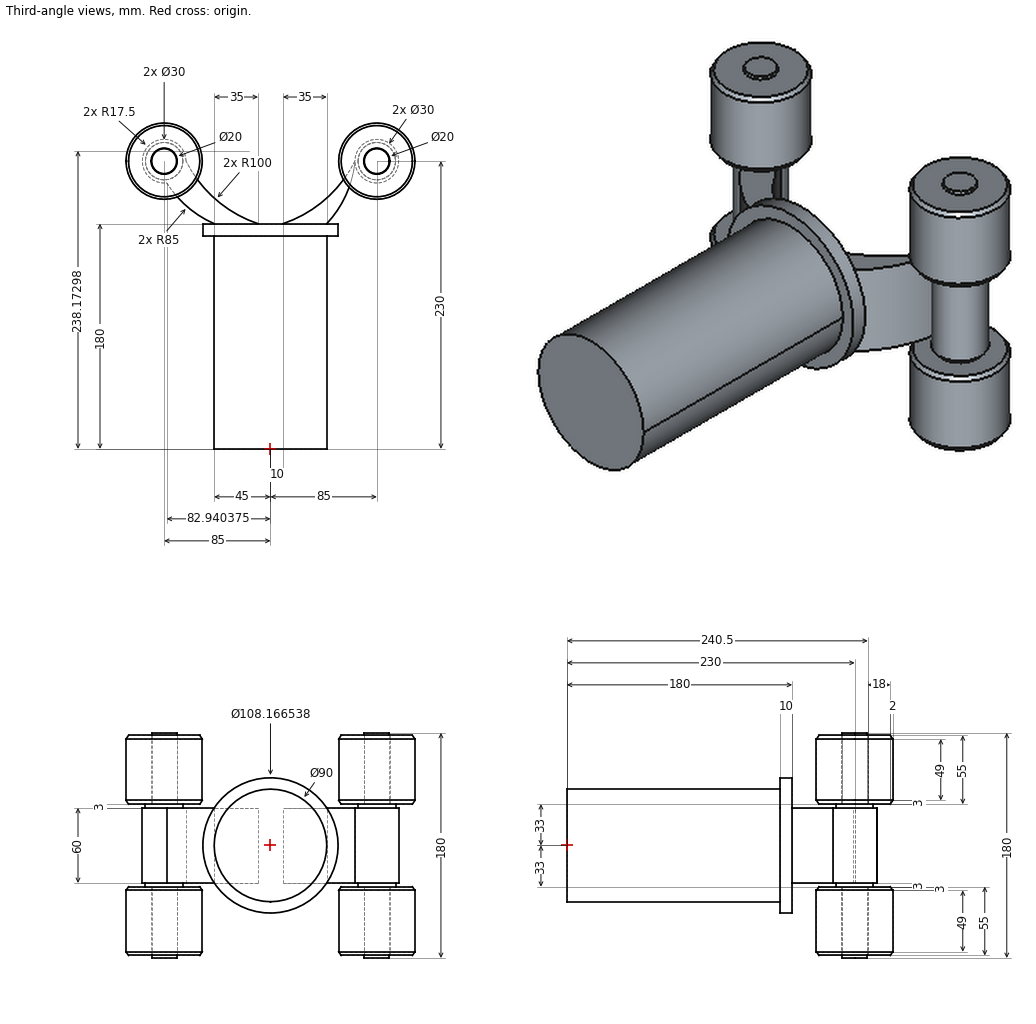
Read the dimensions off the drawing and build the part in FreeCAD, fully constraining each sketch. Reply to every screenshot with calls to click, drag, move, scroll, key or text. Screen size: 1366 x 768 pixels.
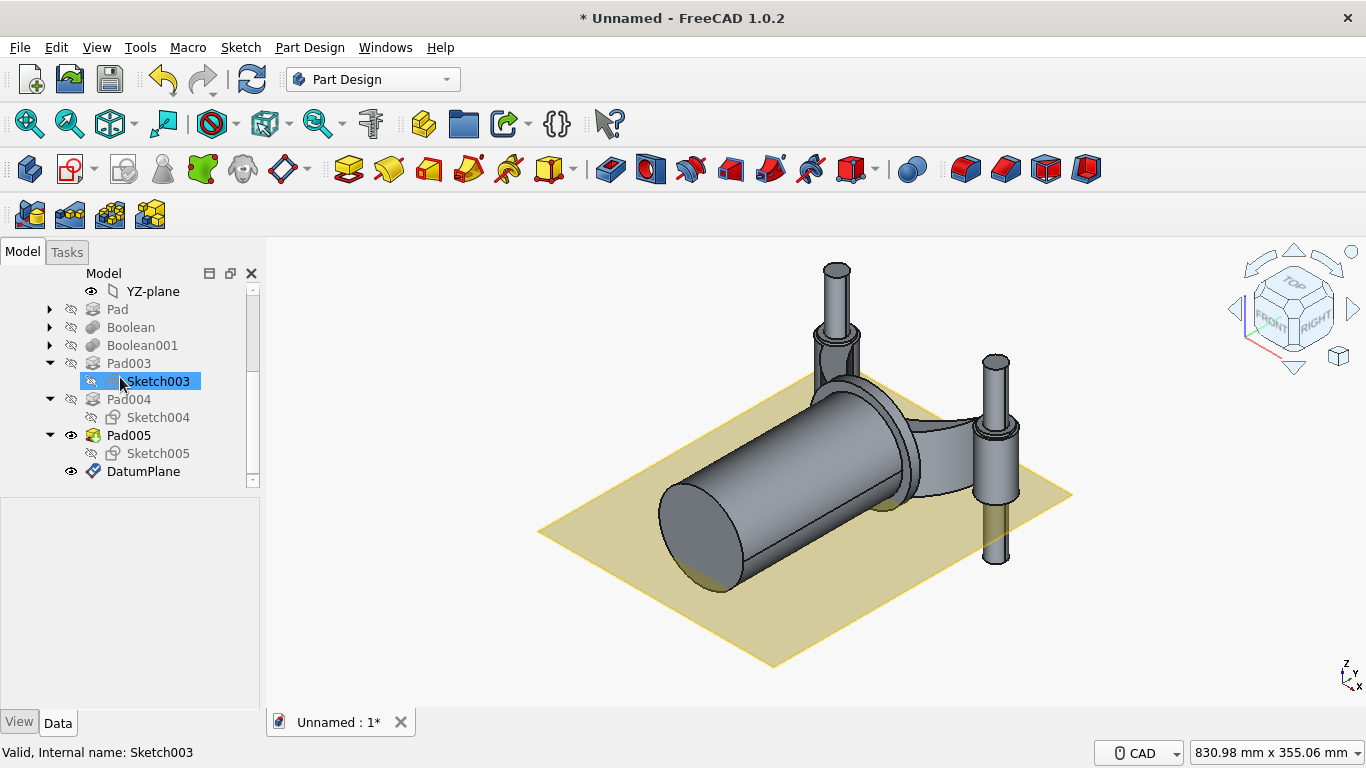
click(116, 471)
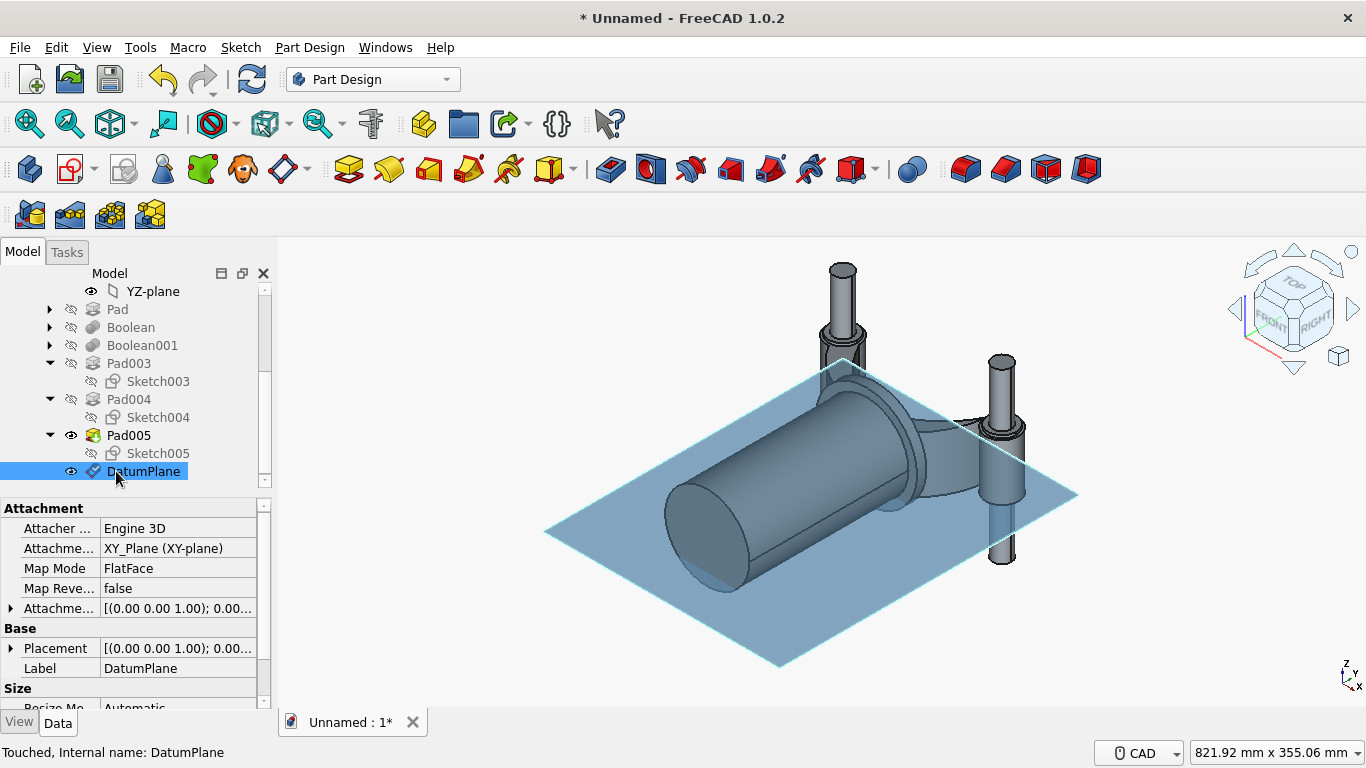
click(70, 170)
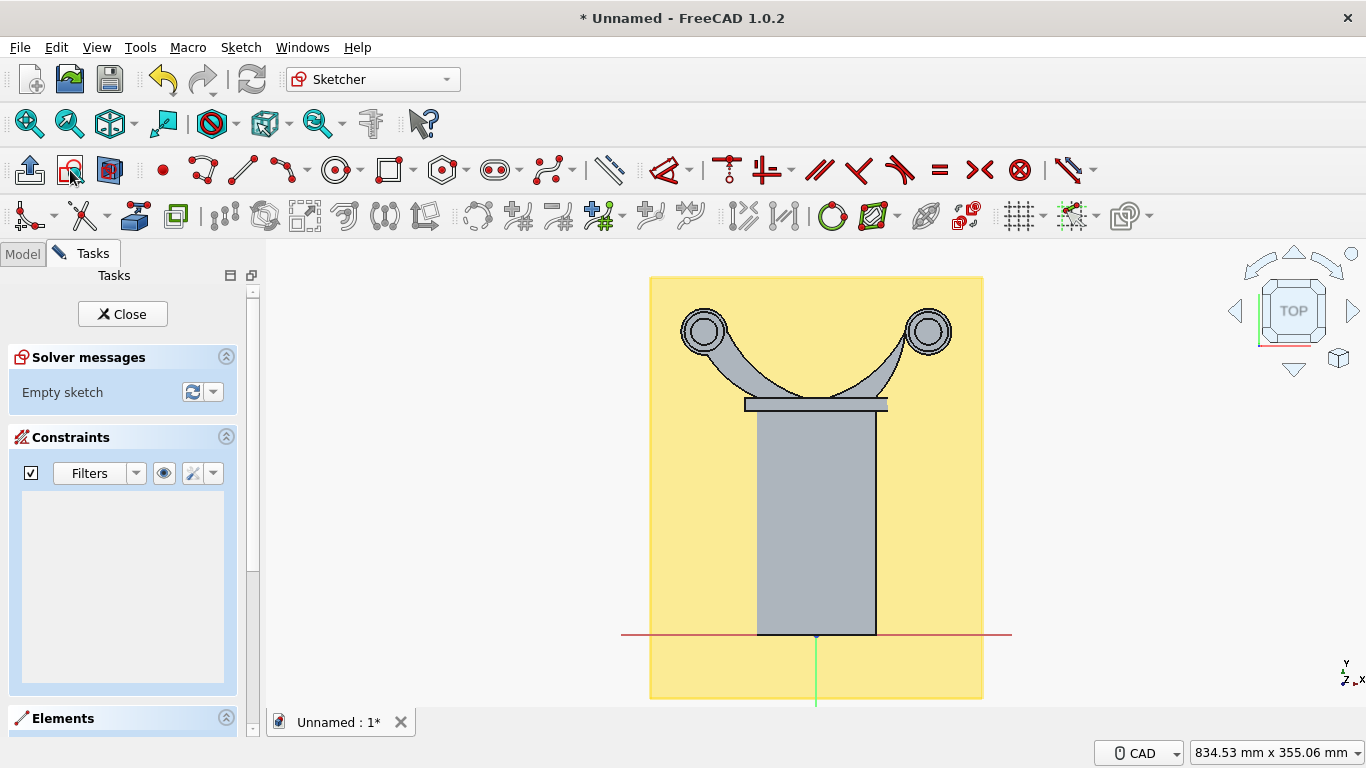
click(110, 170)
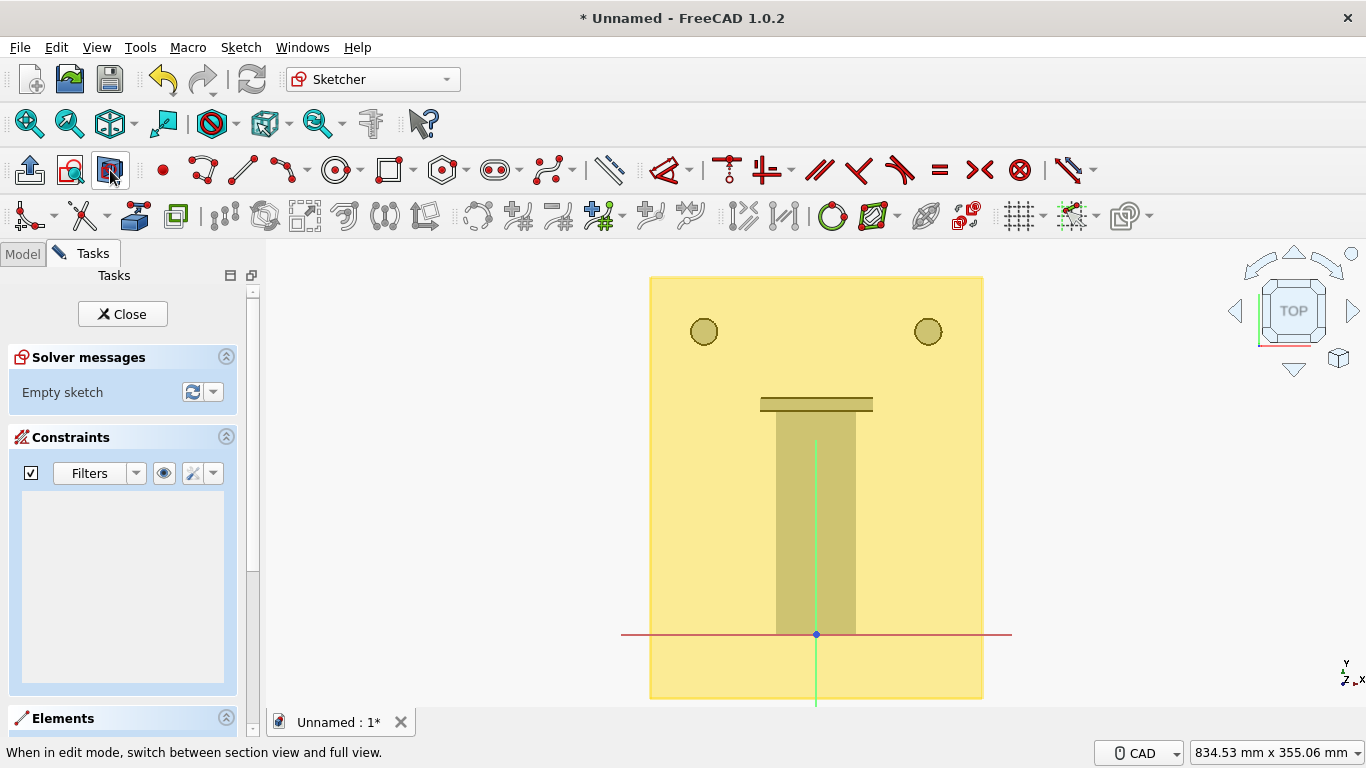
click(336, 170)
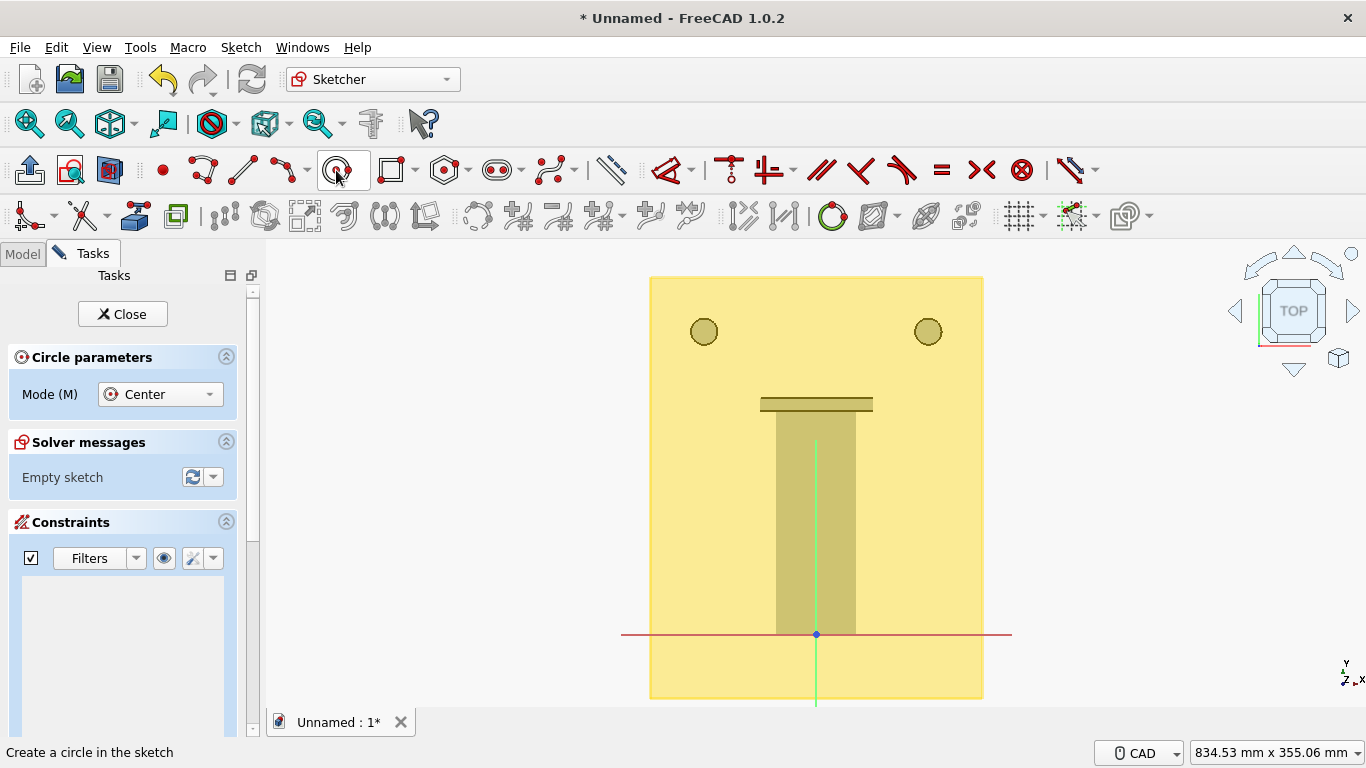
click(928, 332)
click(942, 318)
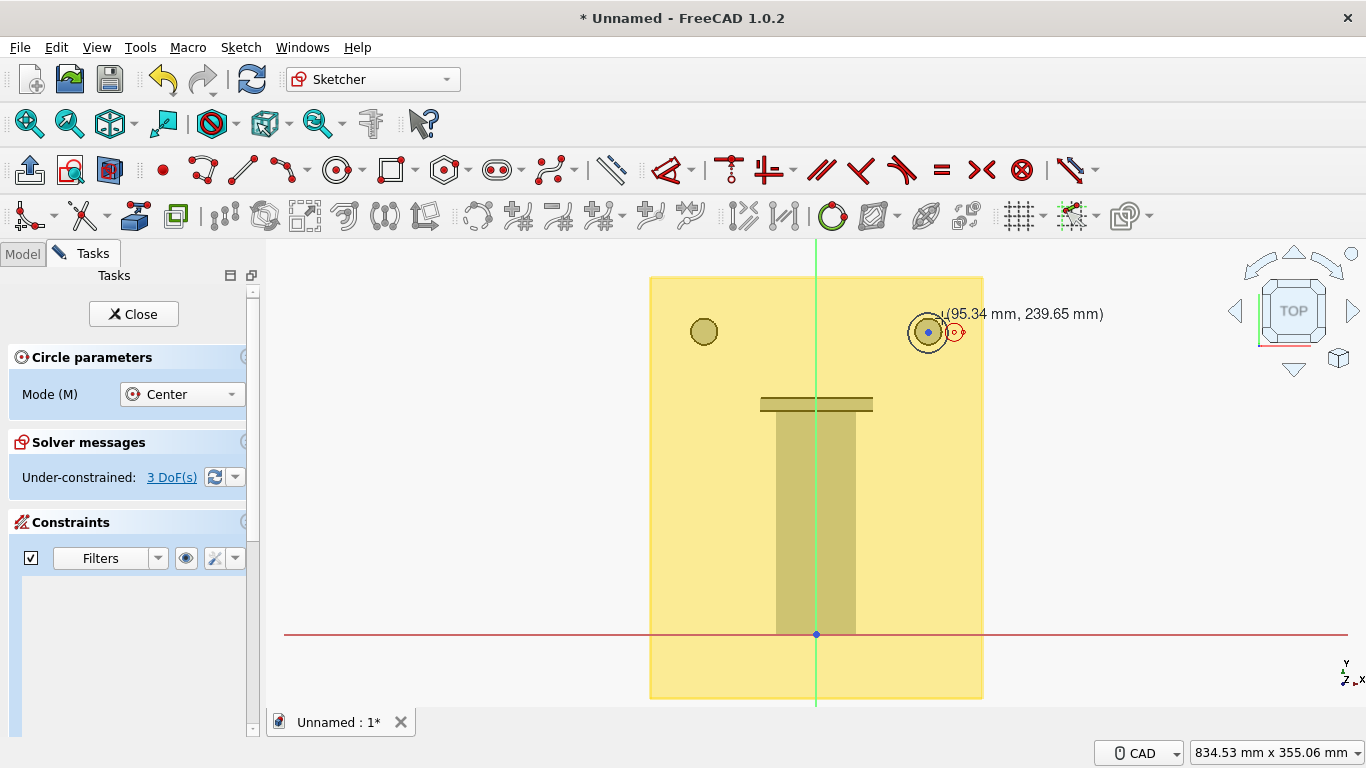
click(704, 332)
click(718, 318)
key(Escape)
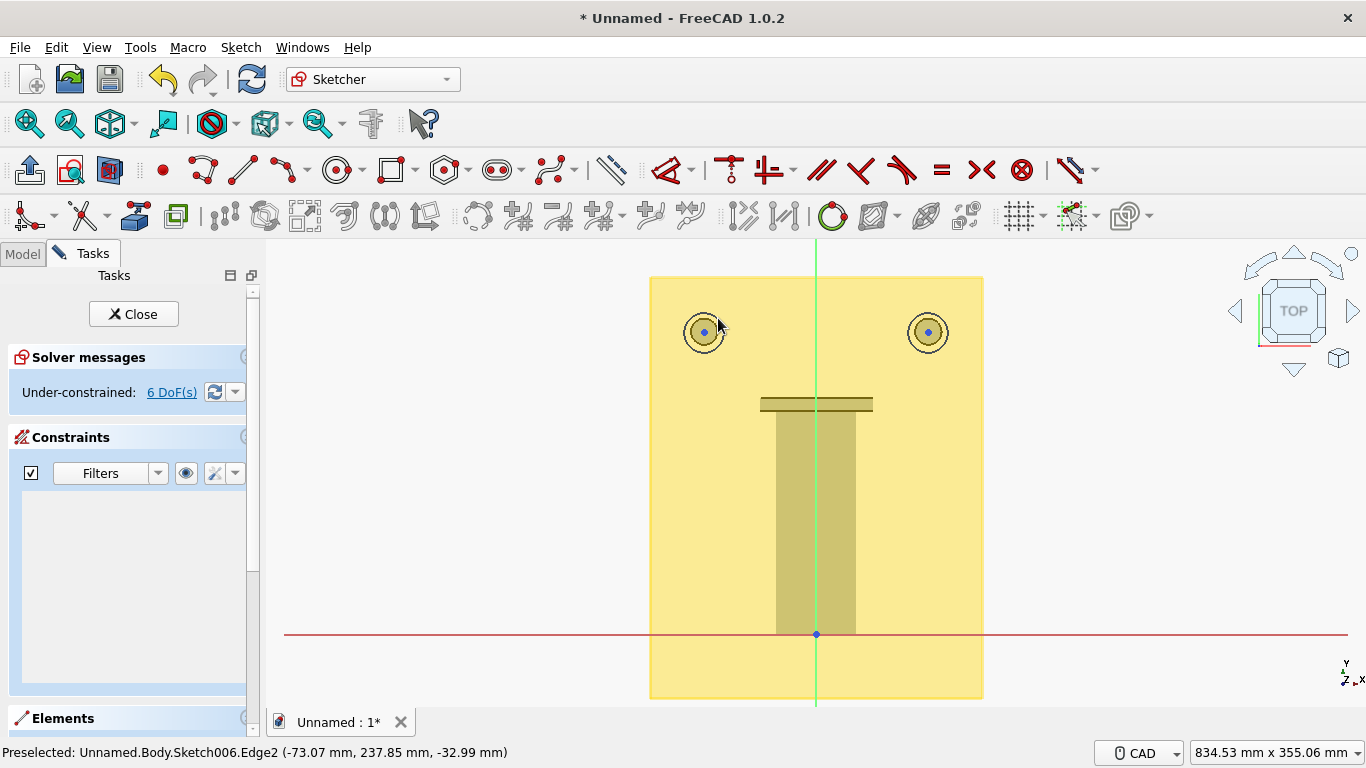
click(942, 319)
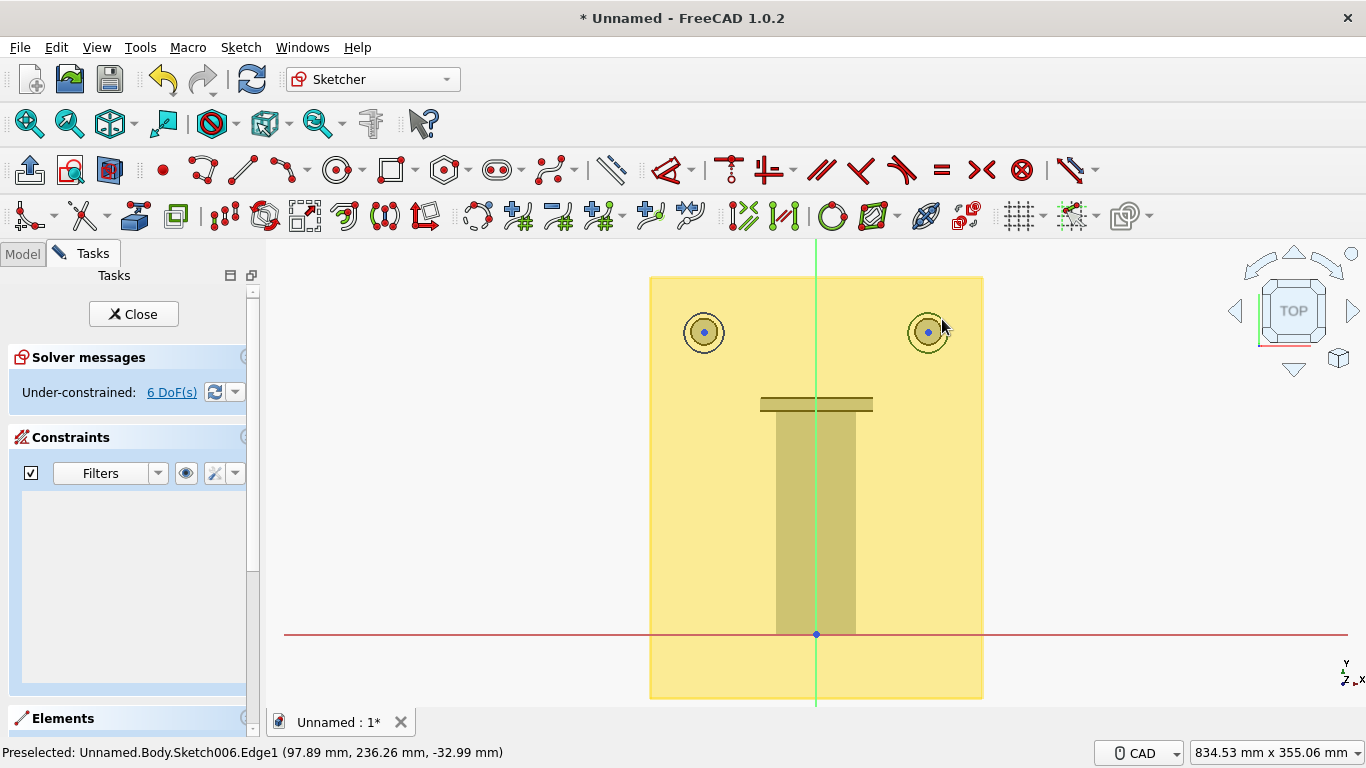
click(718, 319)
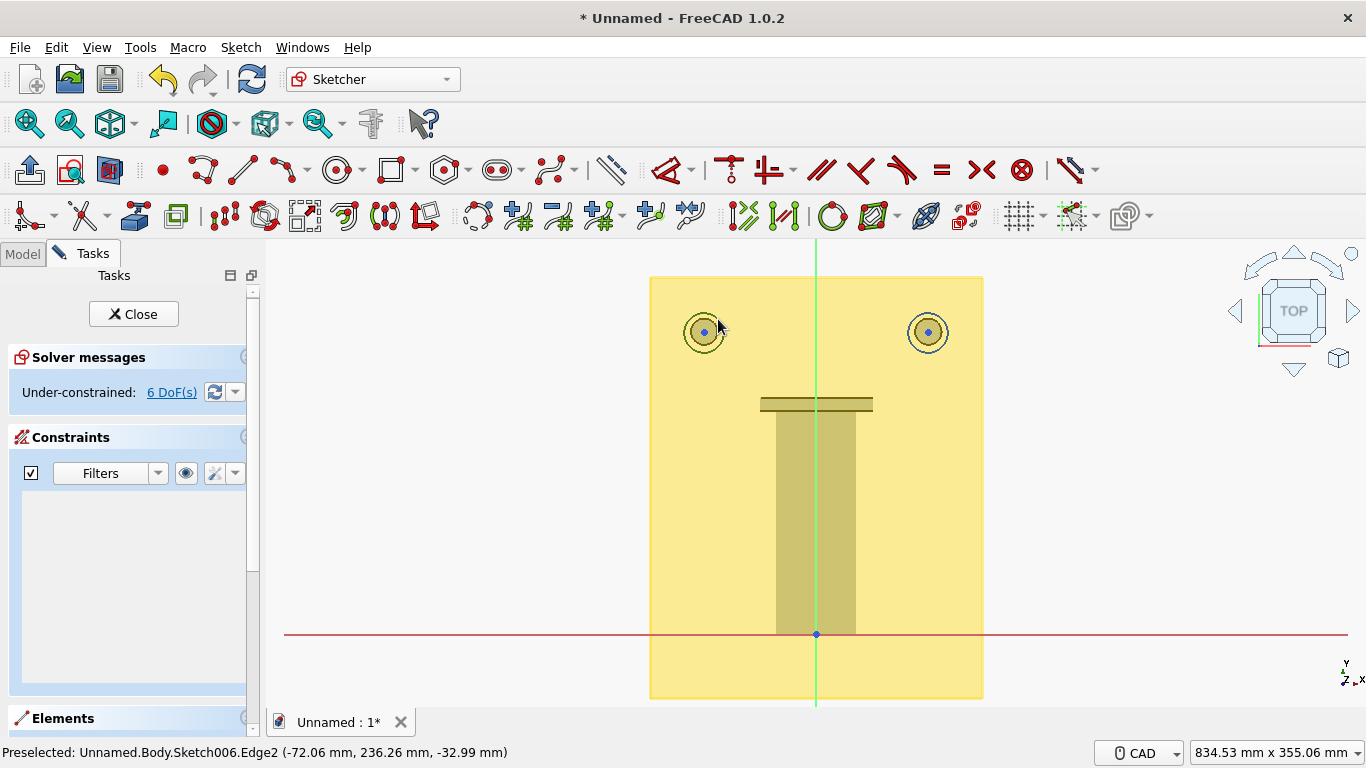
click(942, 170)